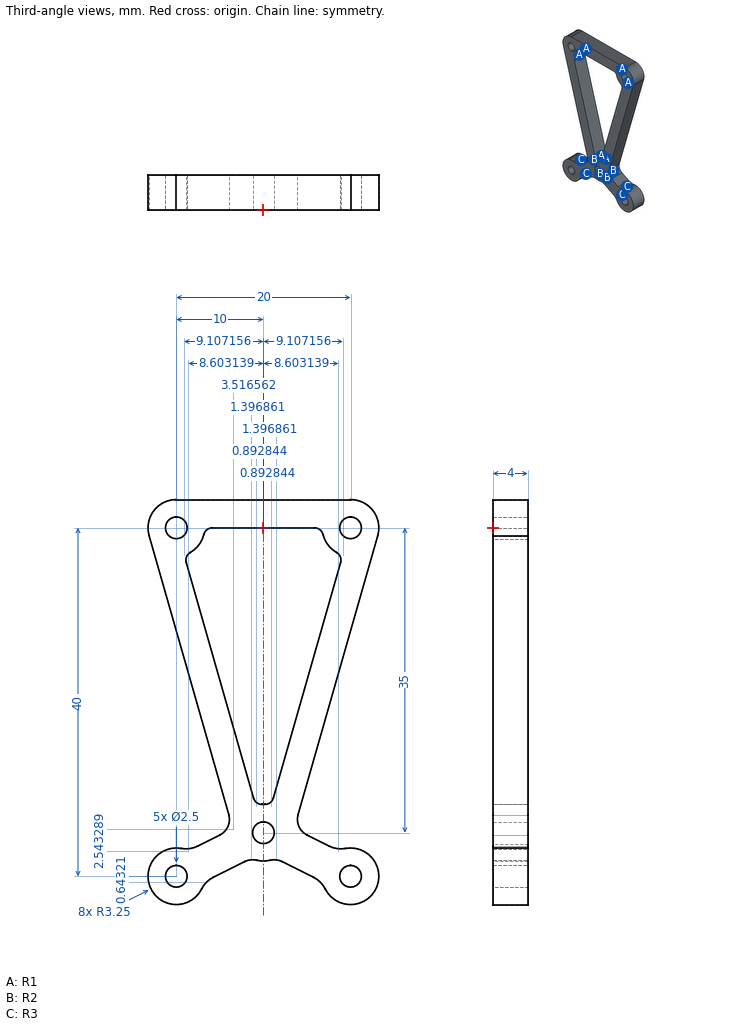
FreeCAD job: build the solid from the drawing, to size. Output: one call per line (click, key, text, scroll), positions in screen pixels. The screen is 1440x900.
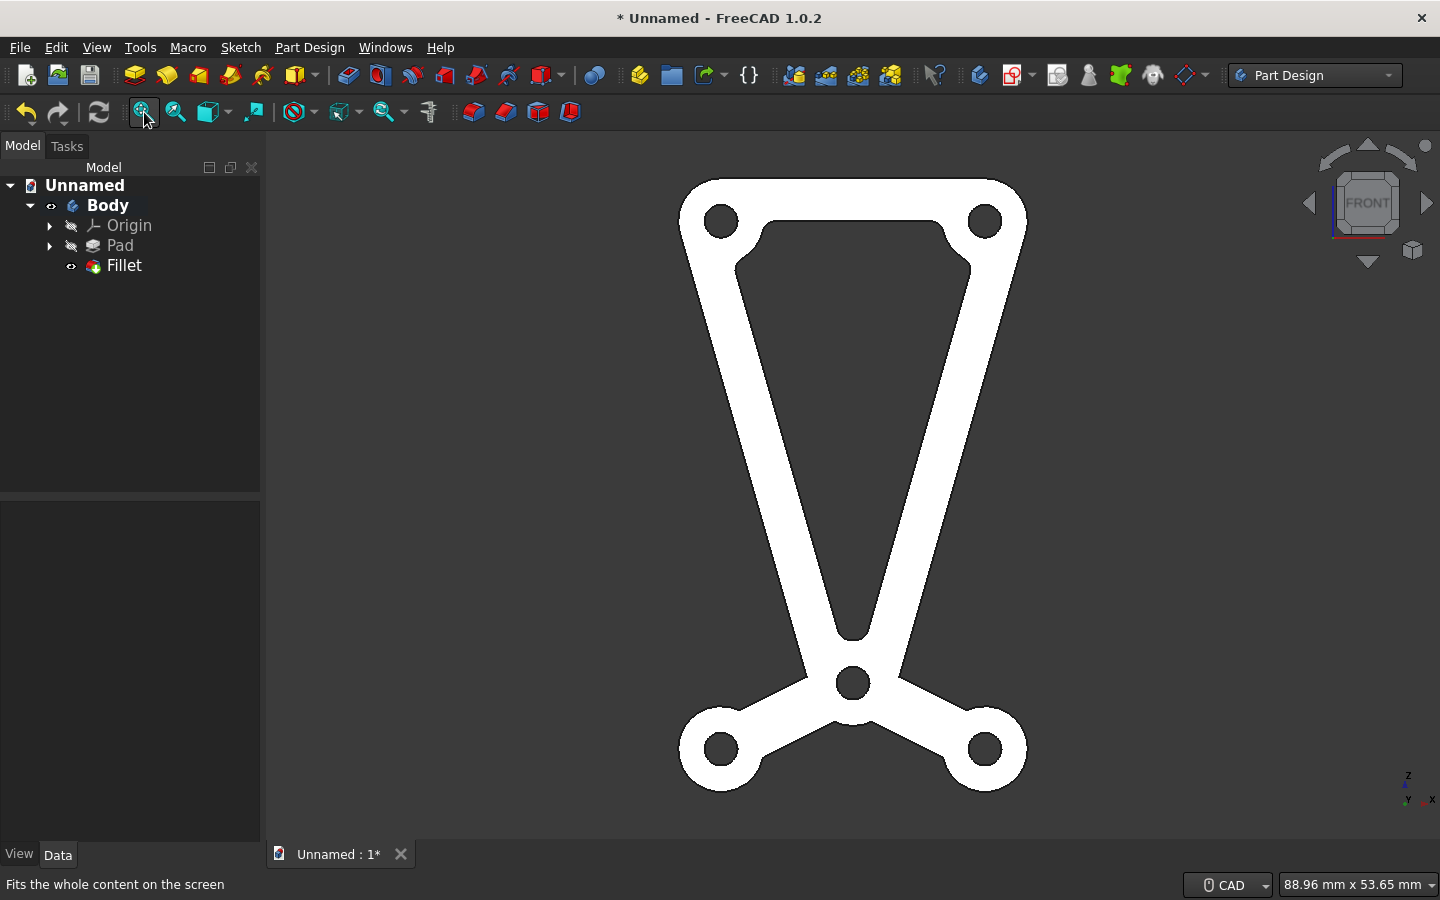
key(3)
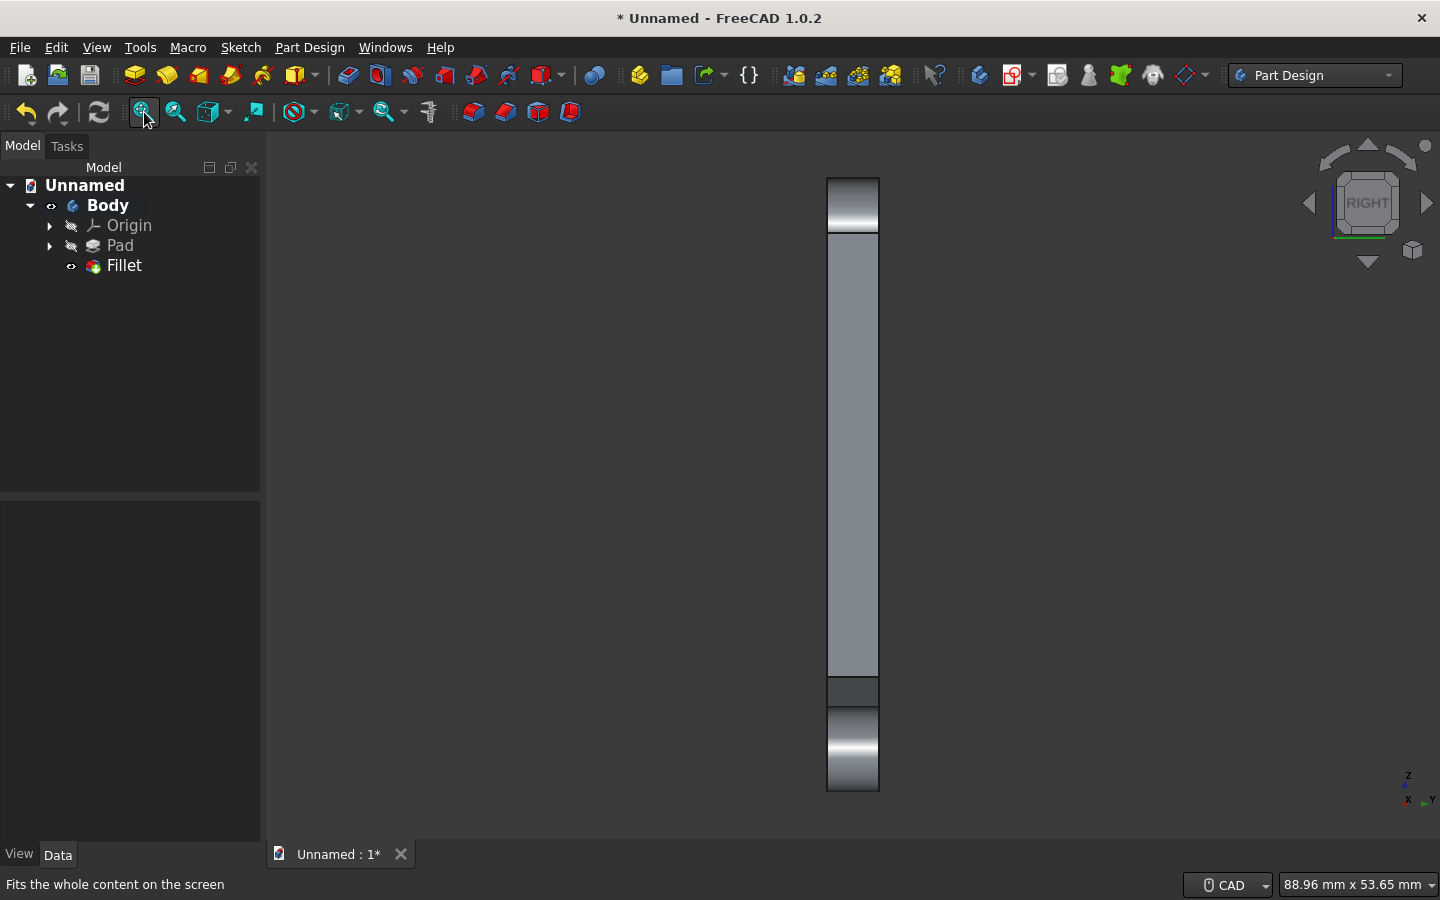
key(5)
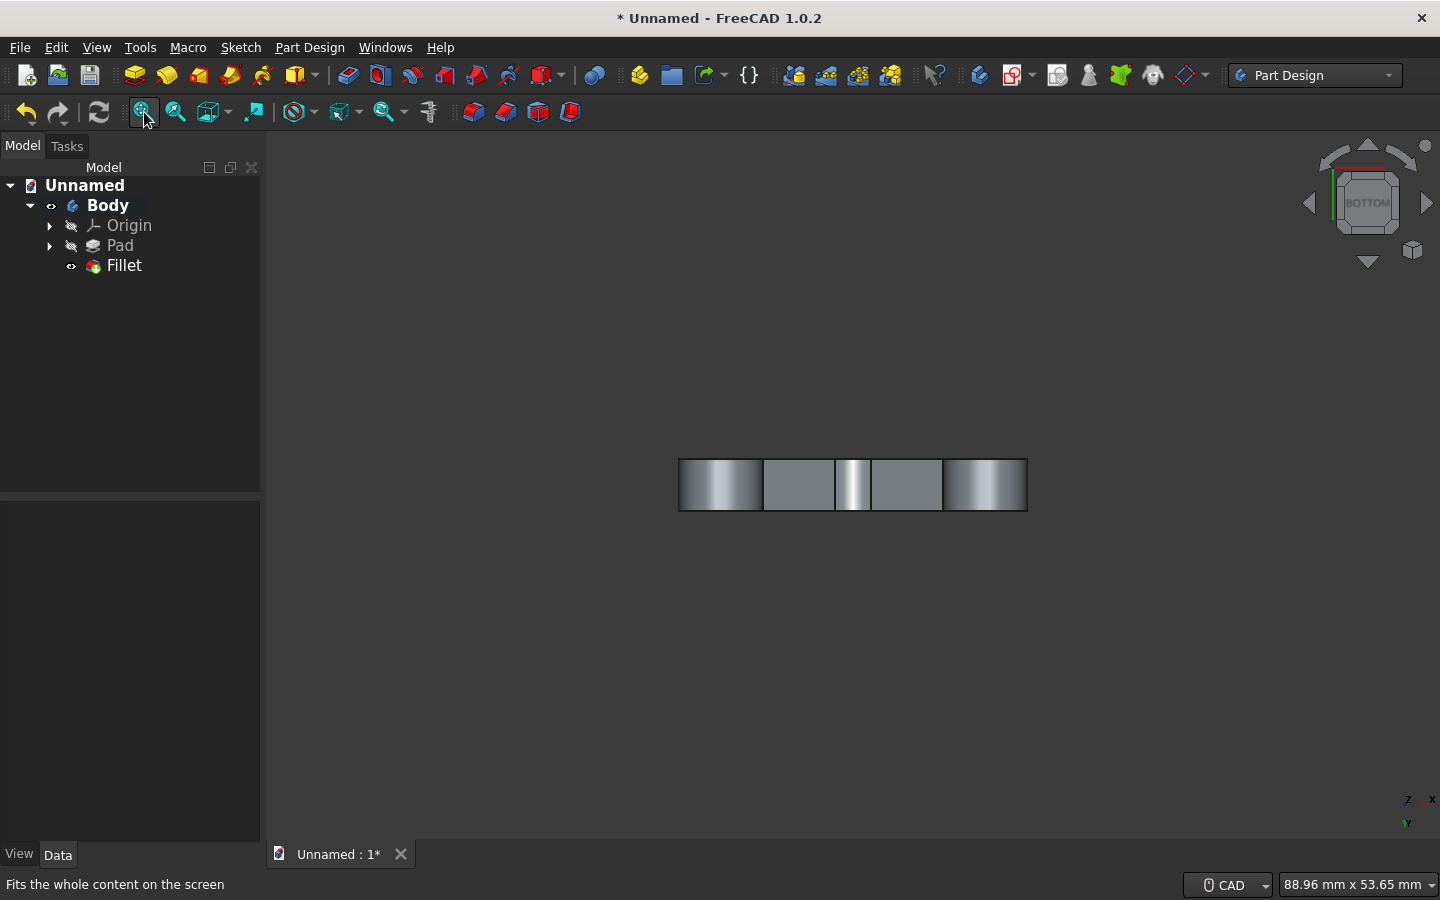
key(v)
key(f)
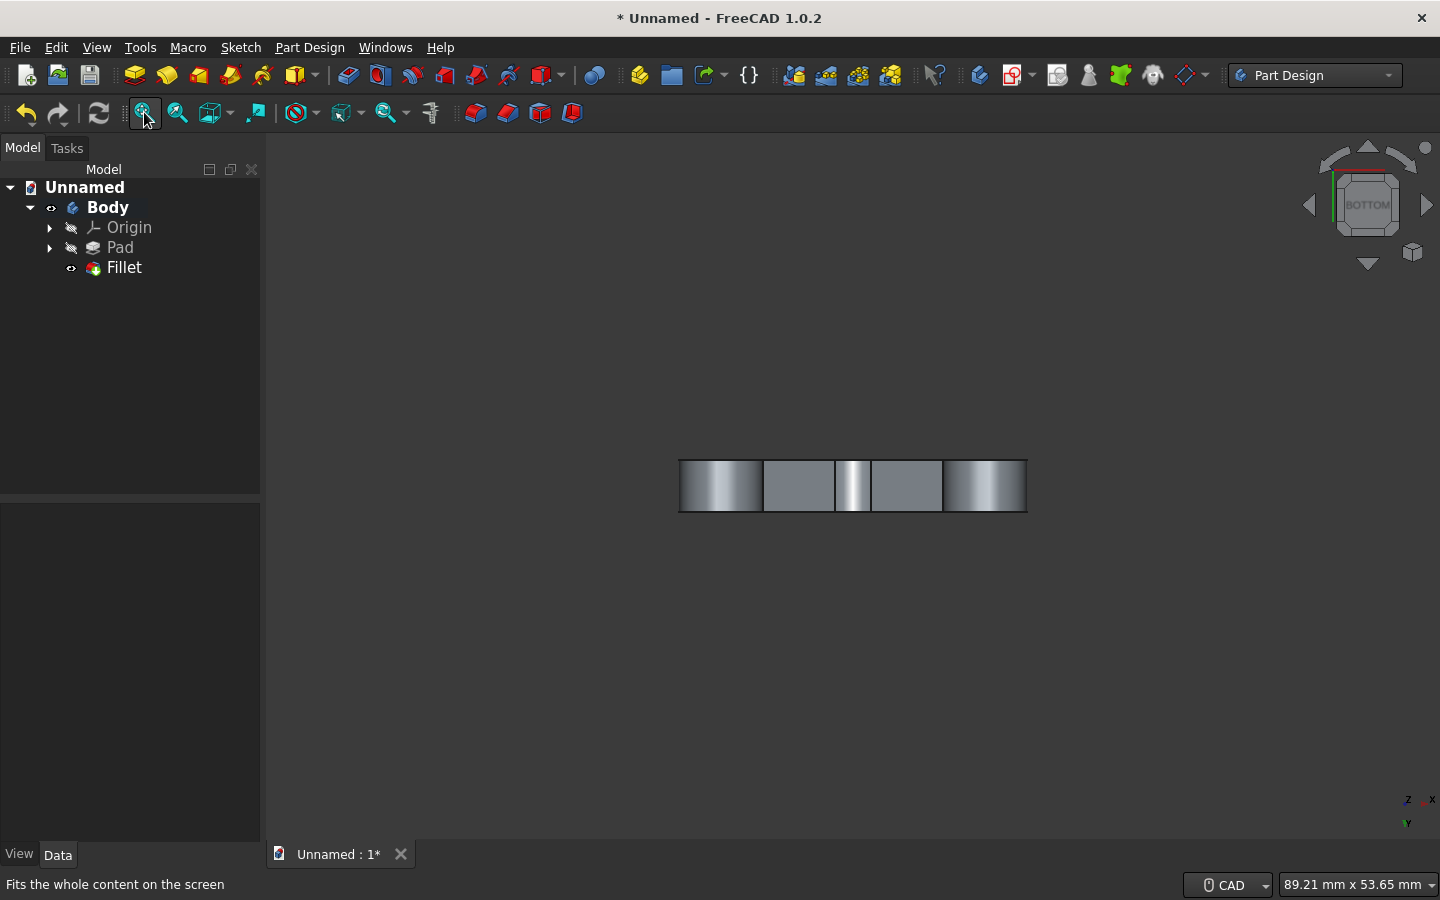
key(4)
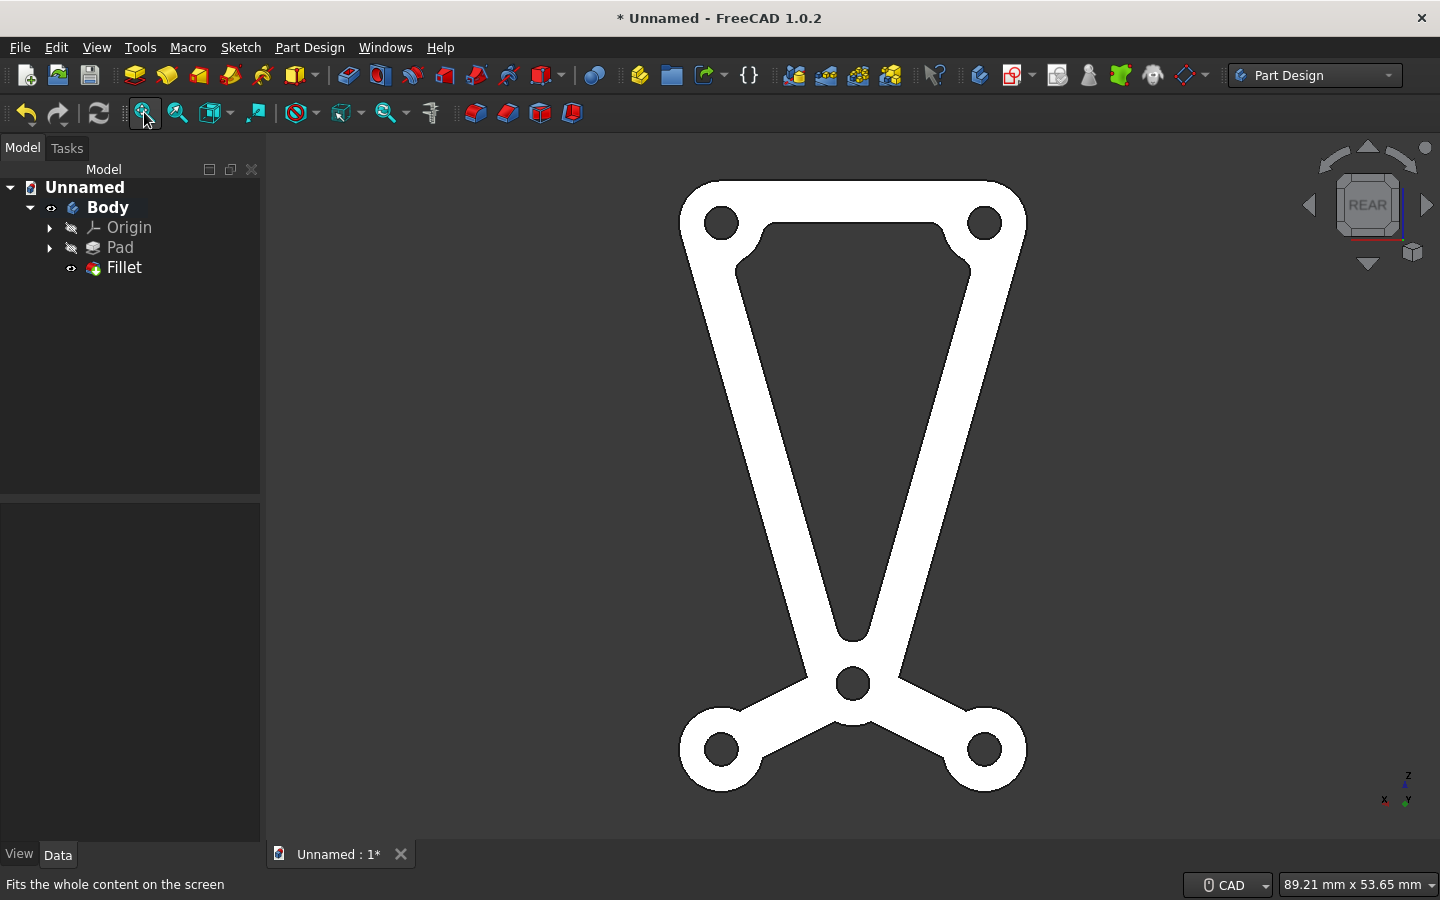
key(6)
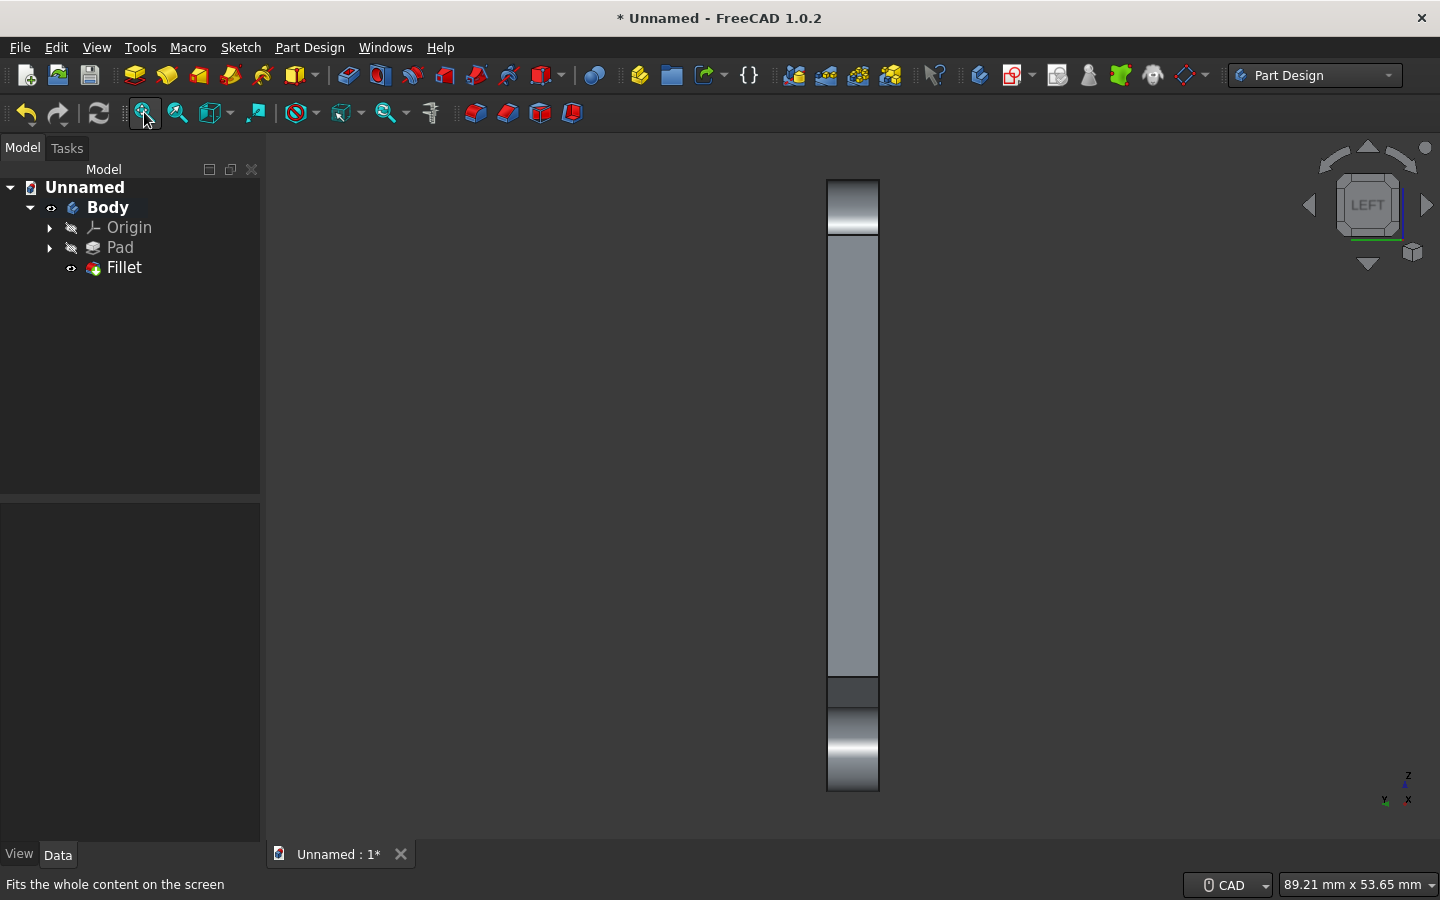
key(v)
key(3)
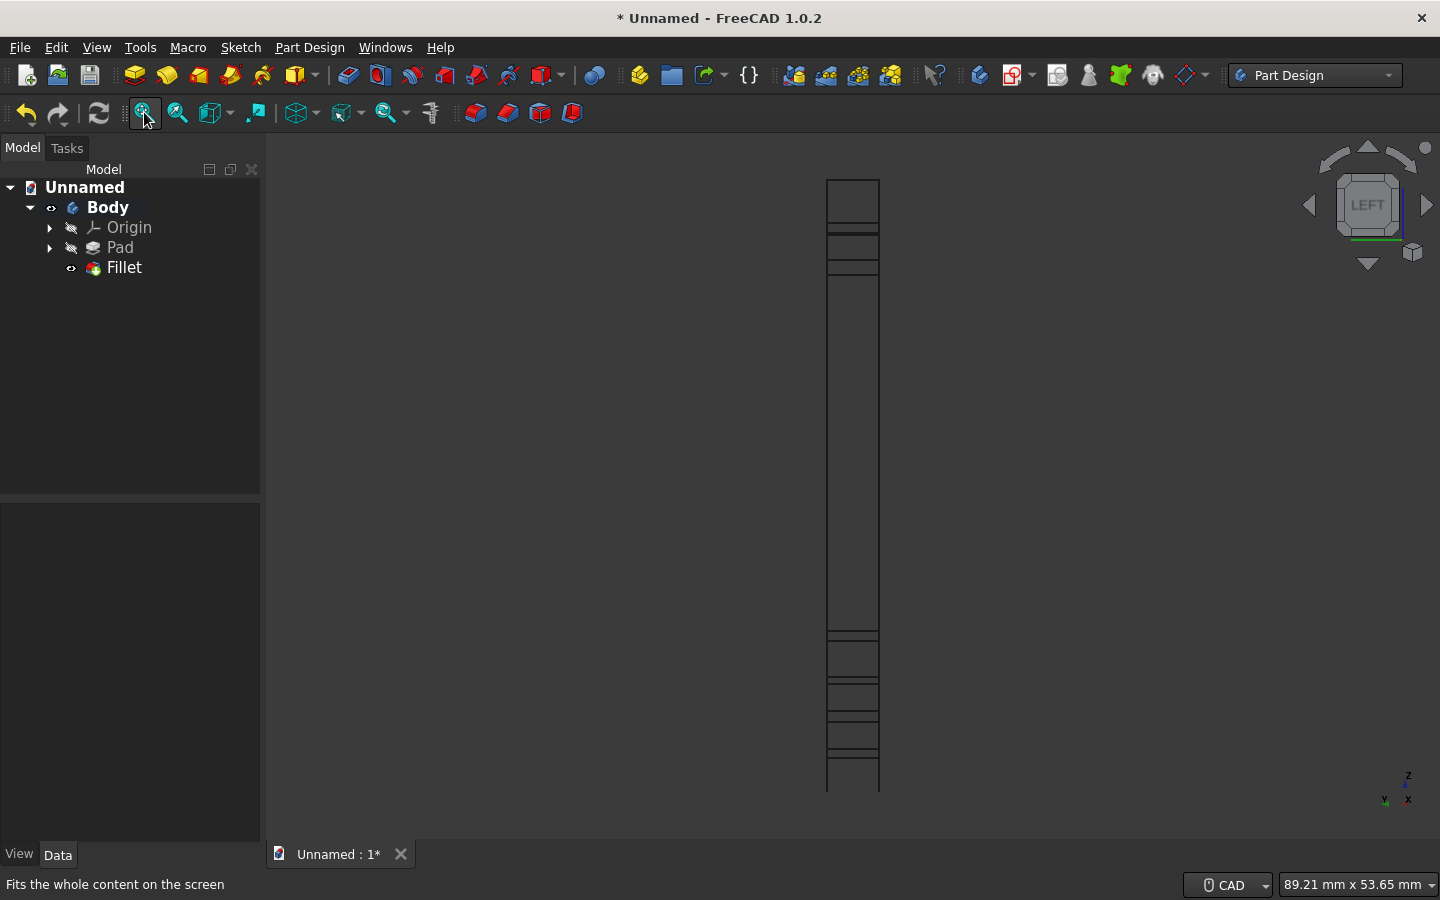
key(0)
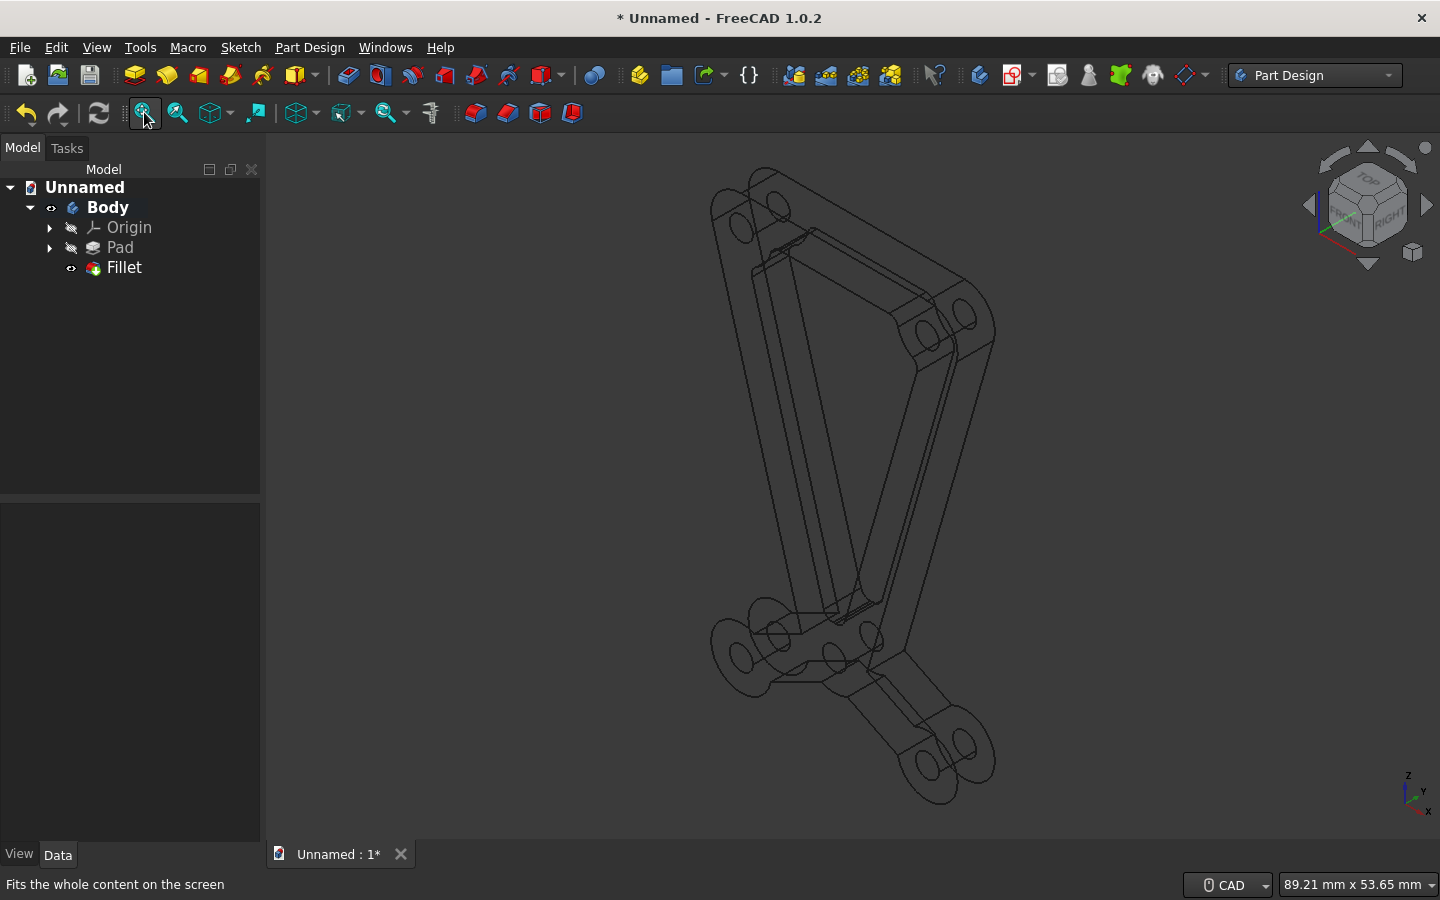
click(820, 622)